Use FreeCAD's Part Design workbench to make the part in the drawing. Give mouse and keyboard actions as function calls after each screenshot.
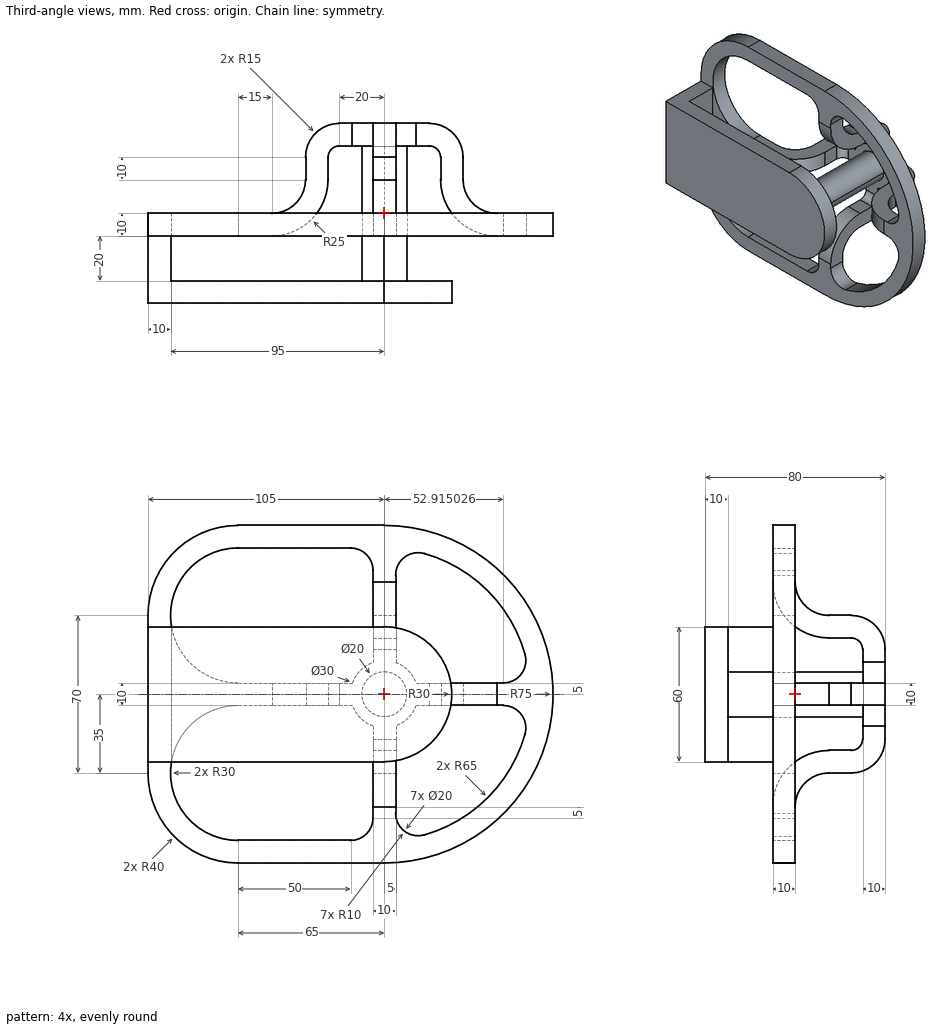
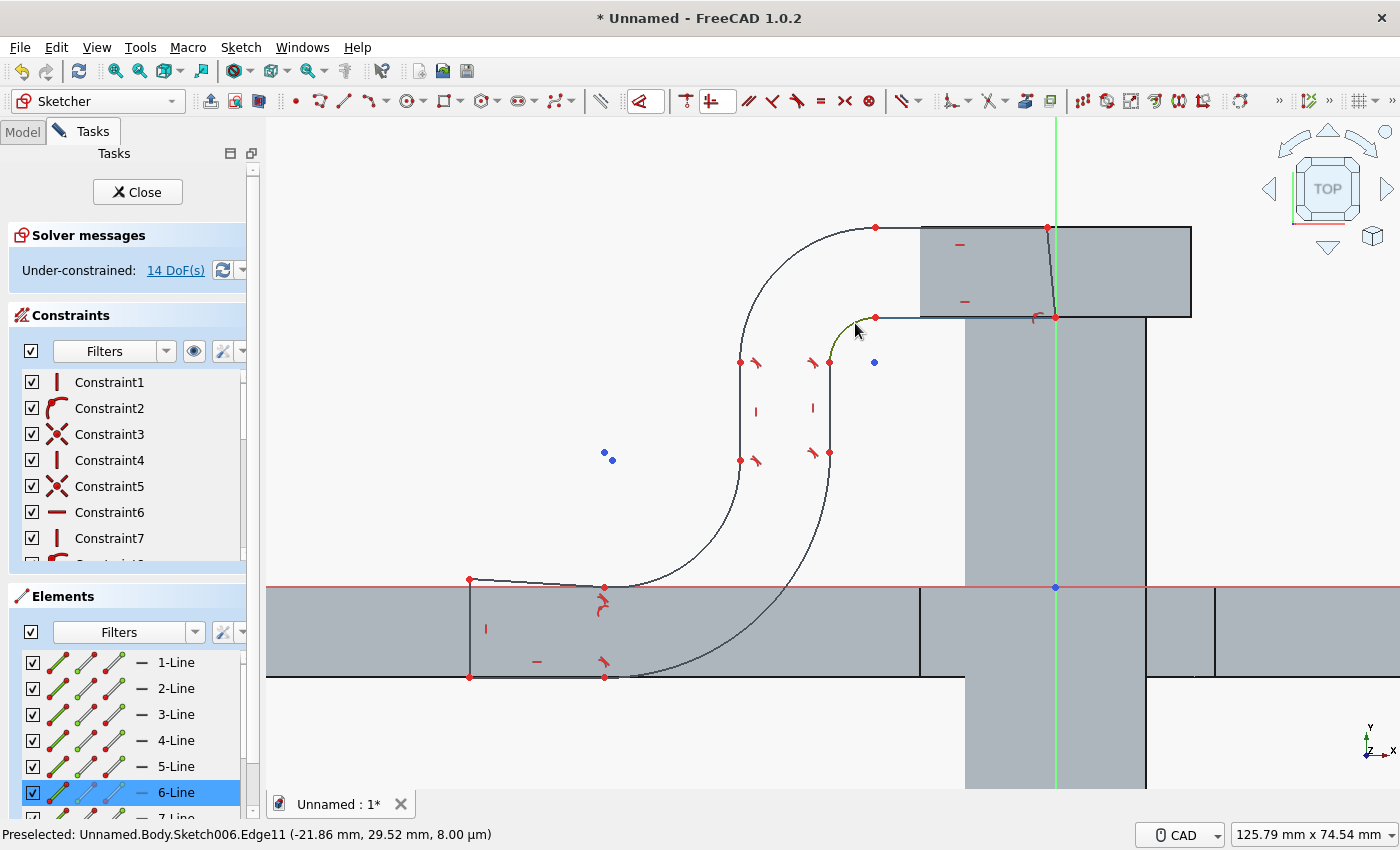
click(798, 102)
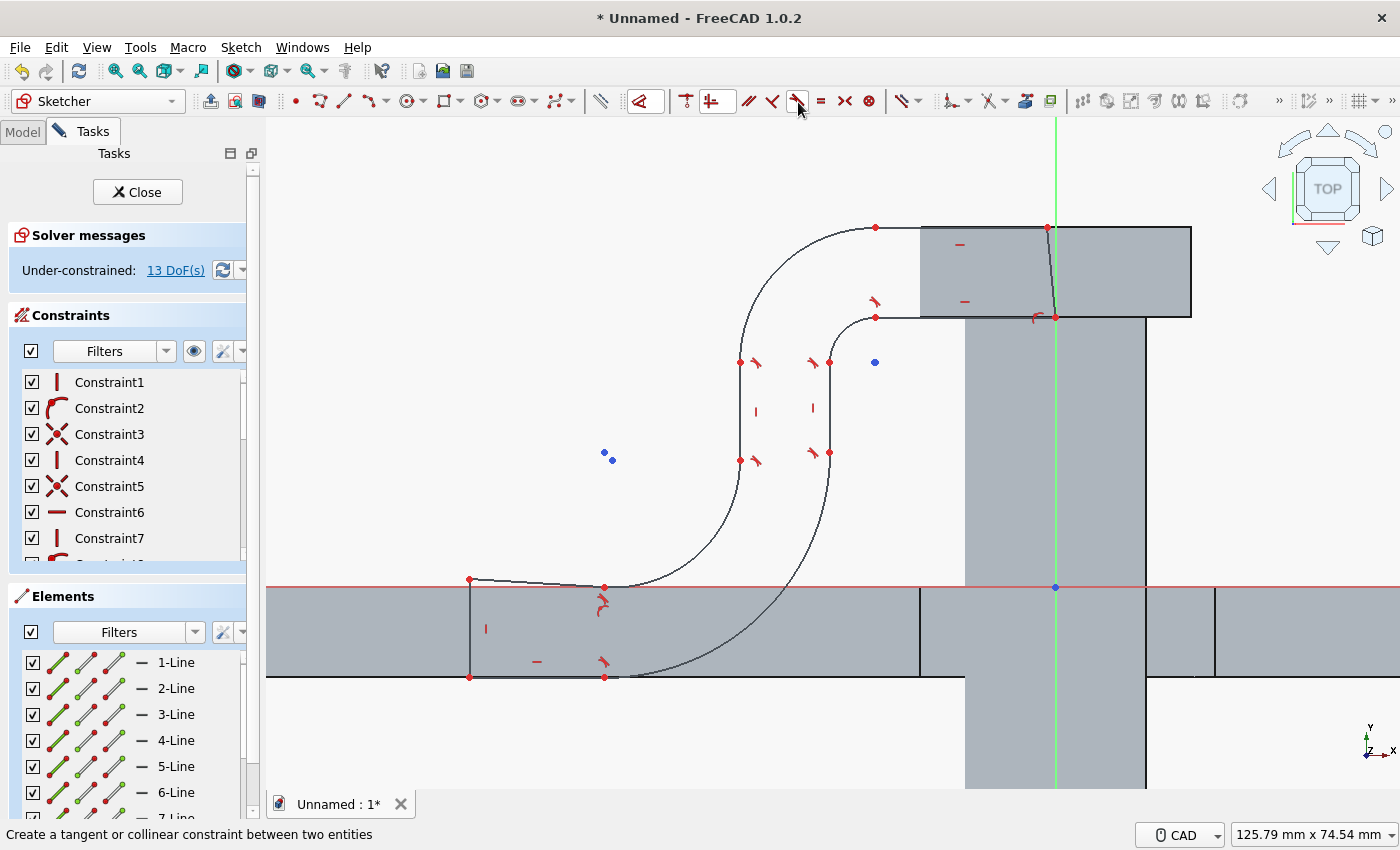
click(995, 228)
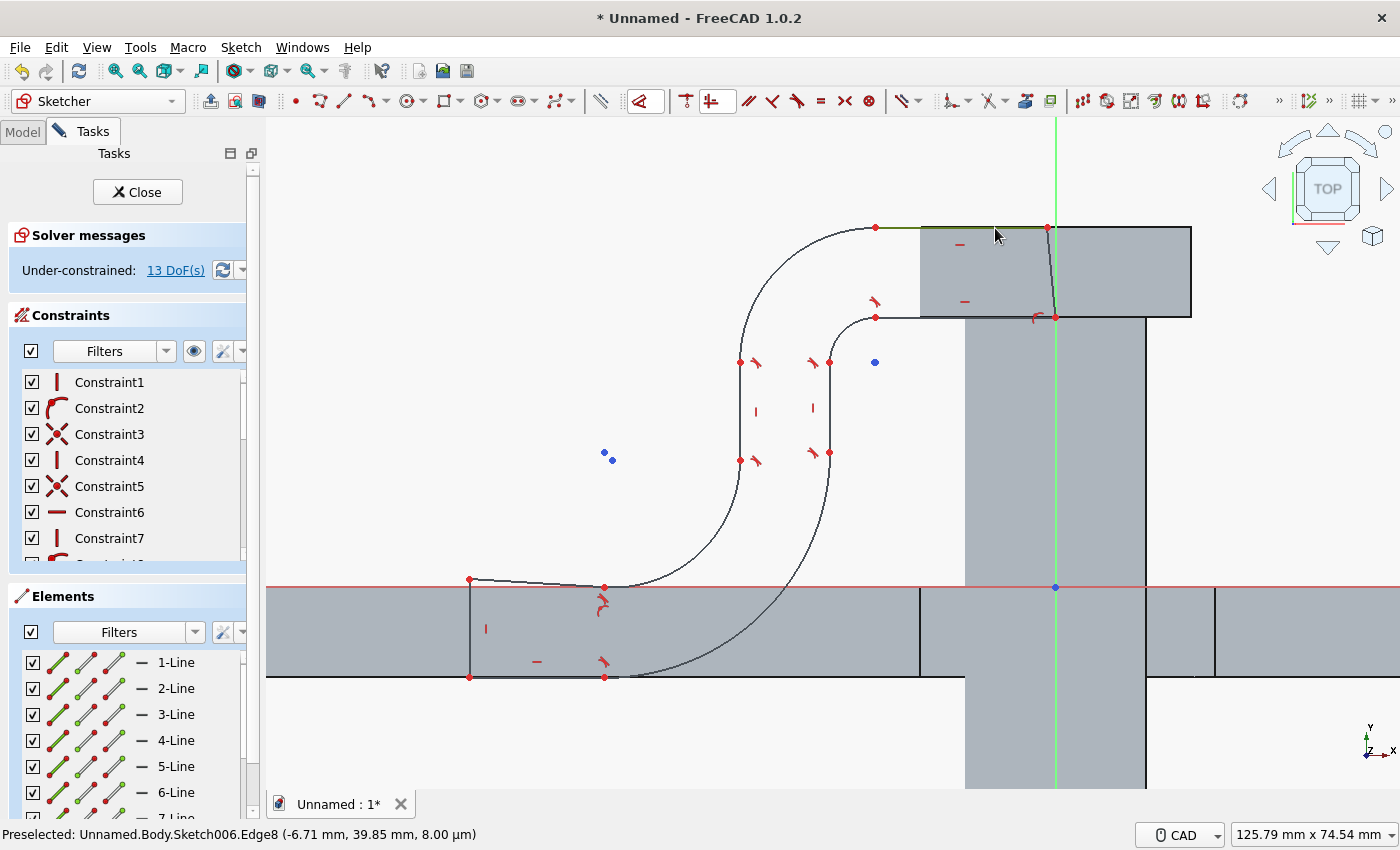
click(814, 243)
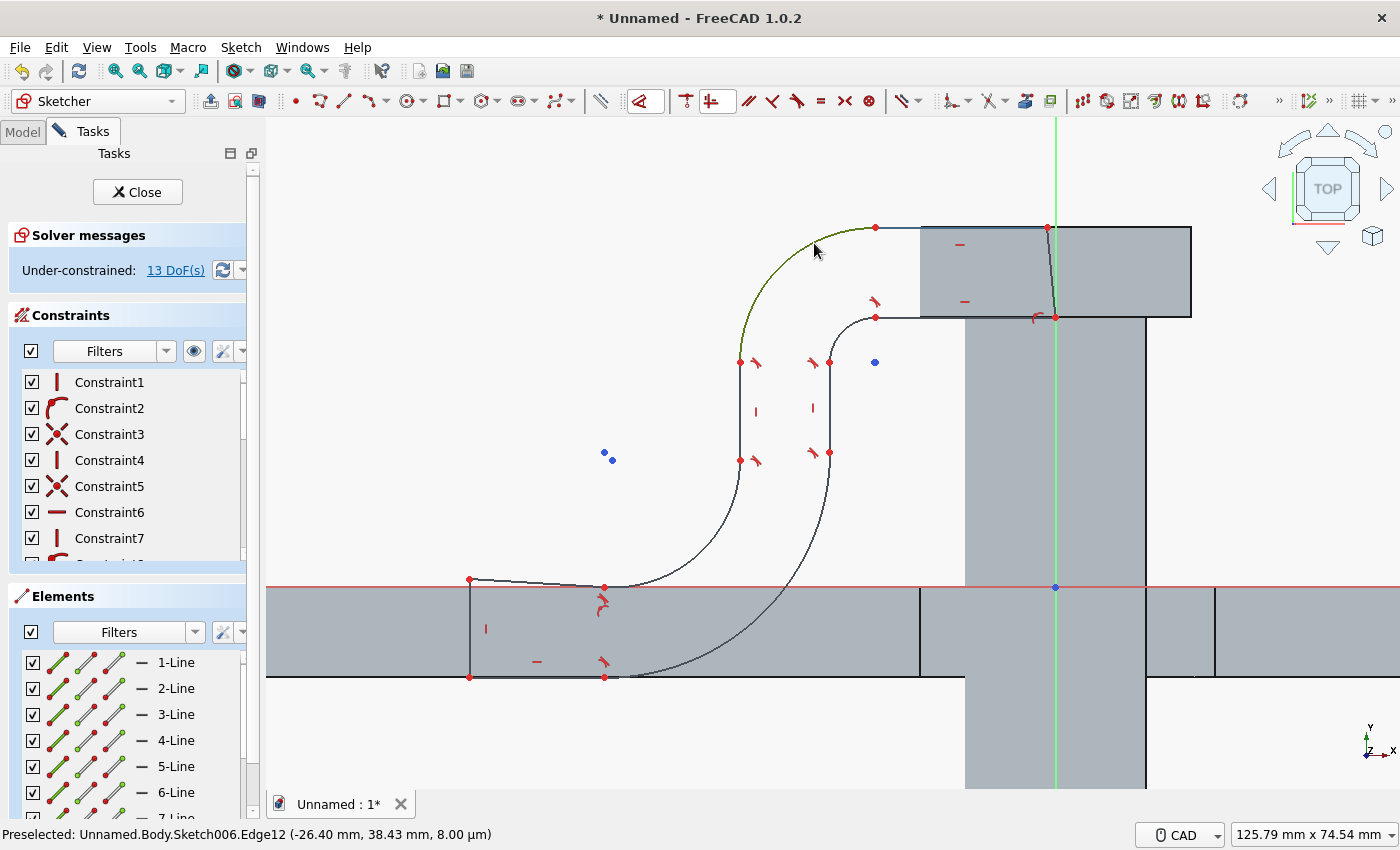
click(798, 102)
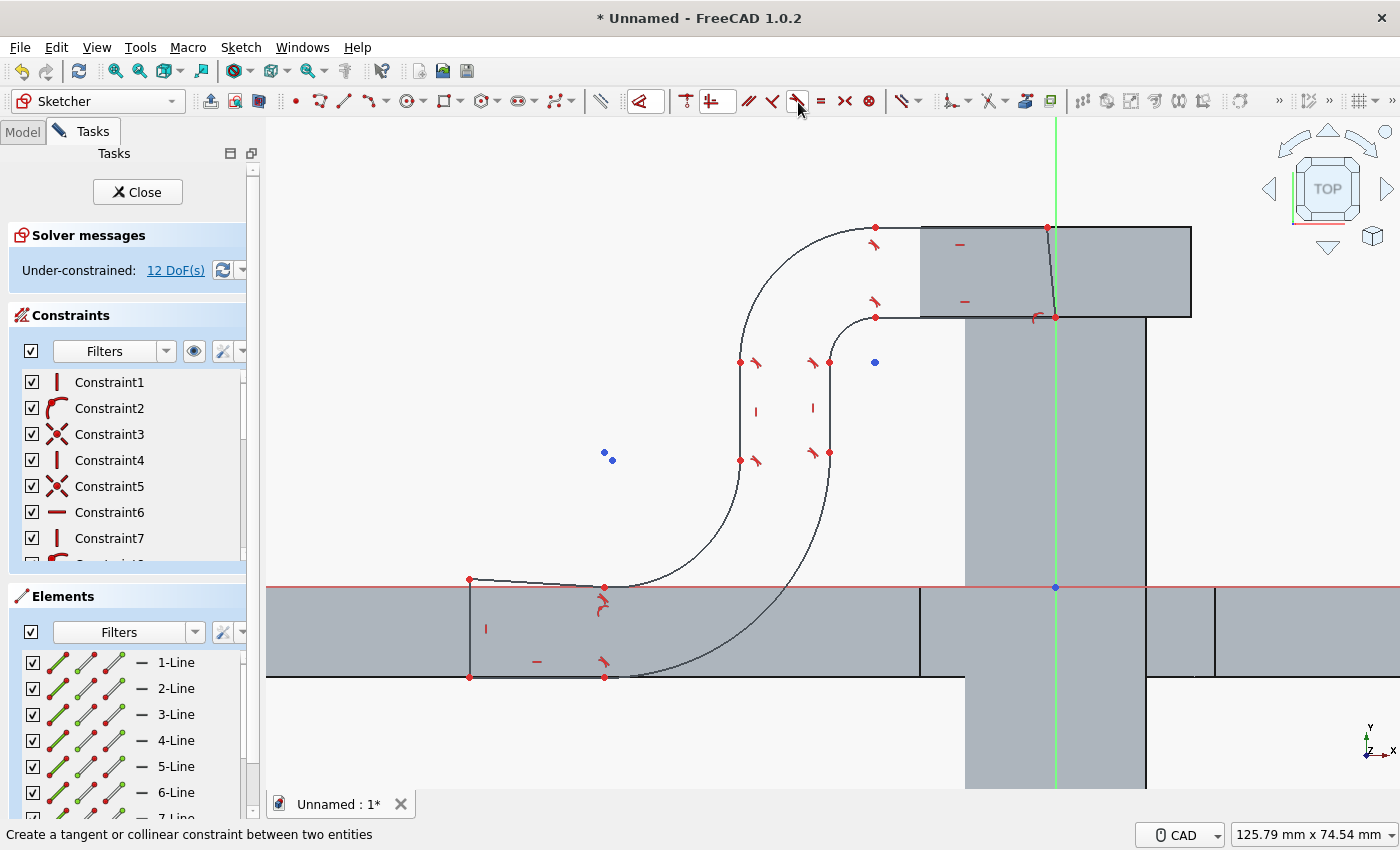
click(564, 585)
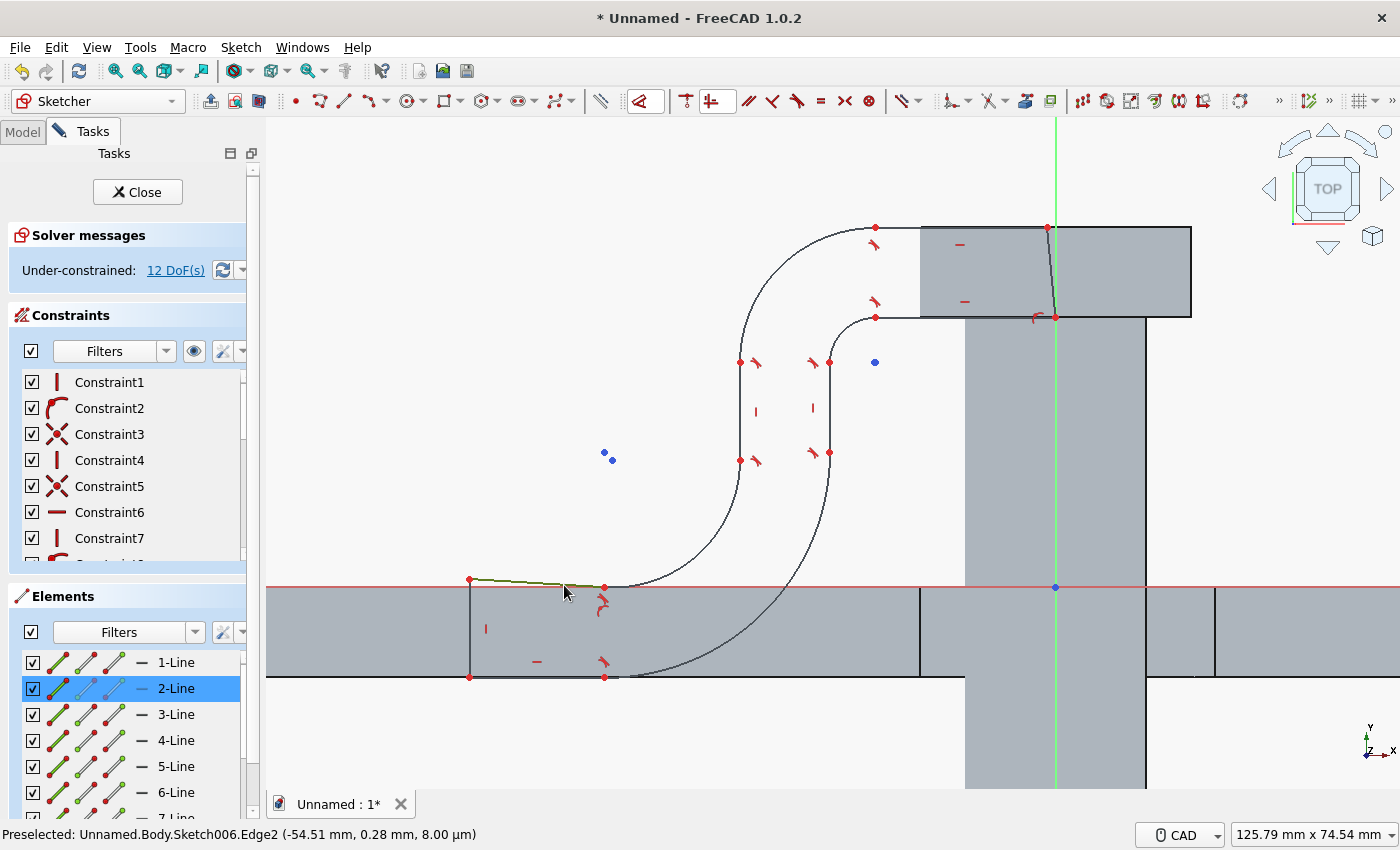
click(730, 102)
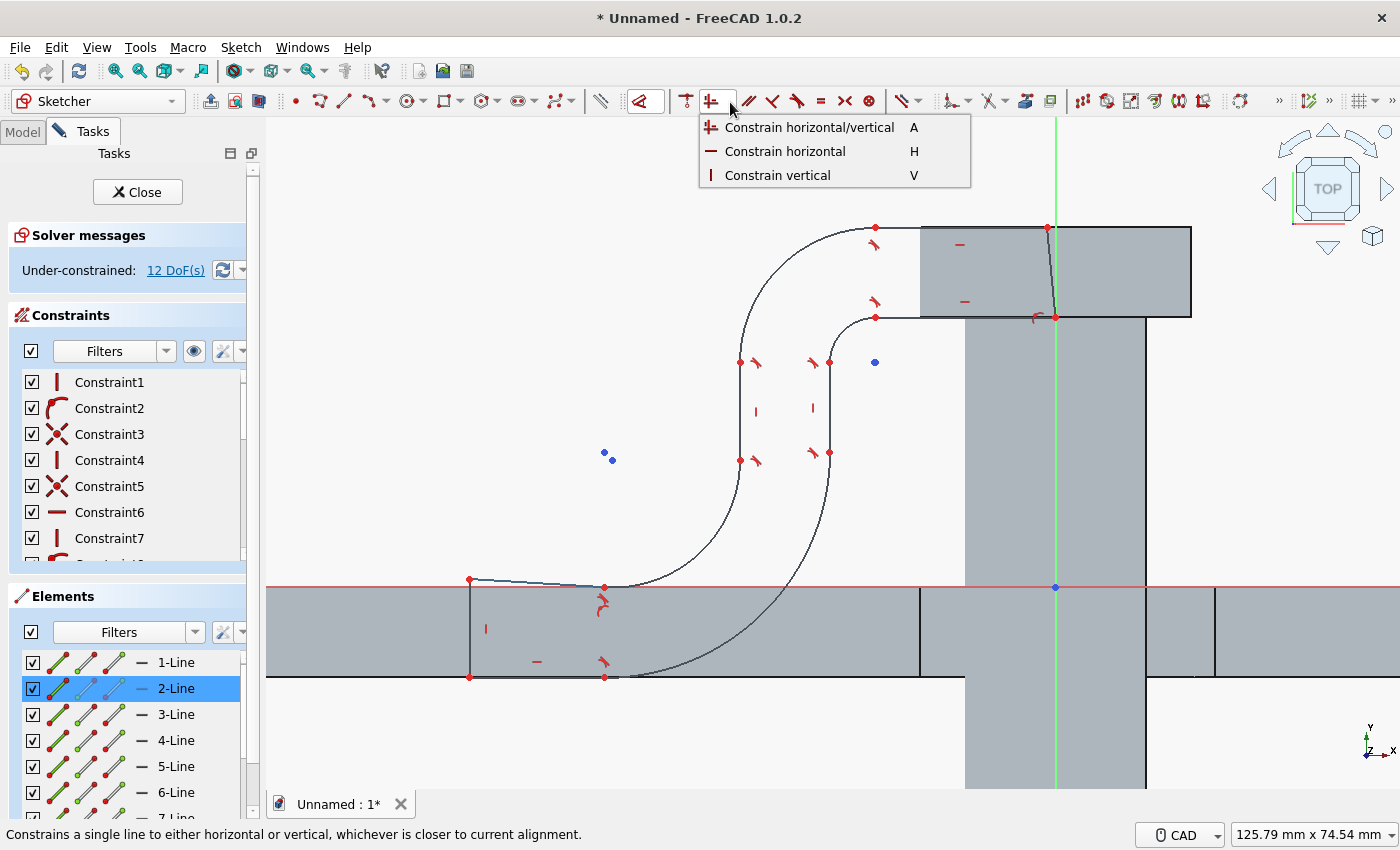
click(835, 151)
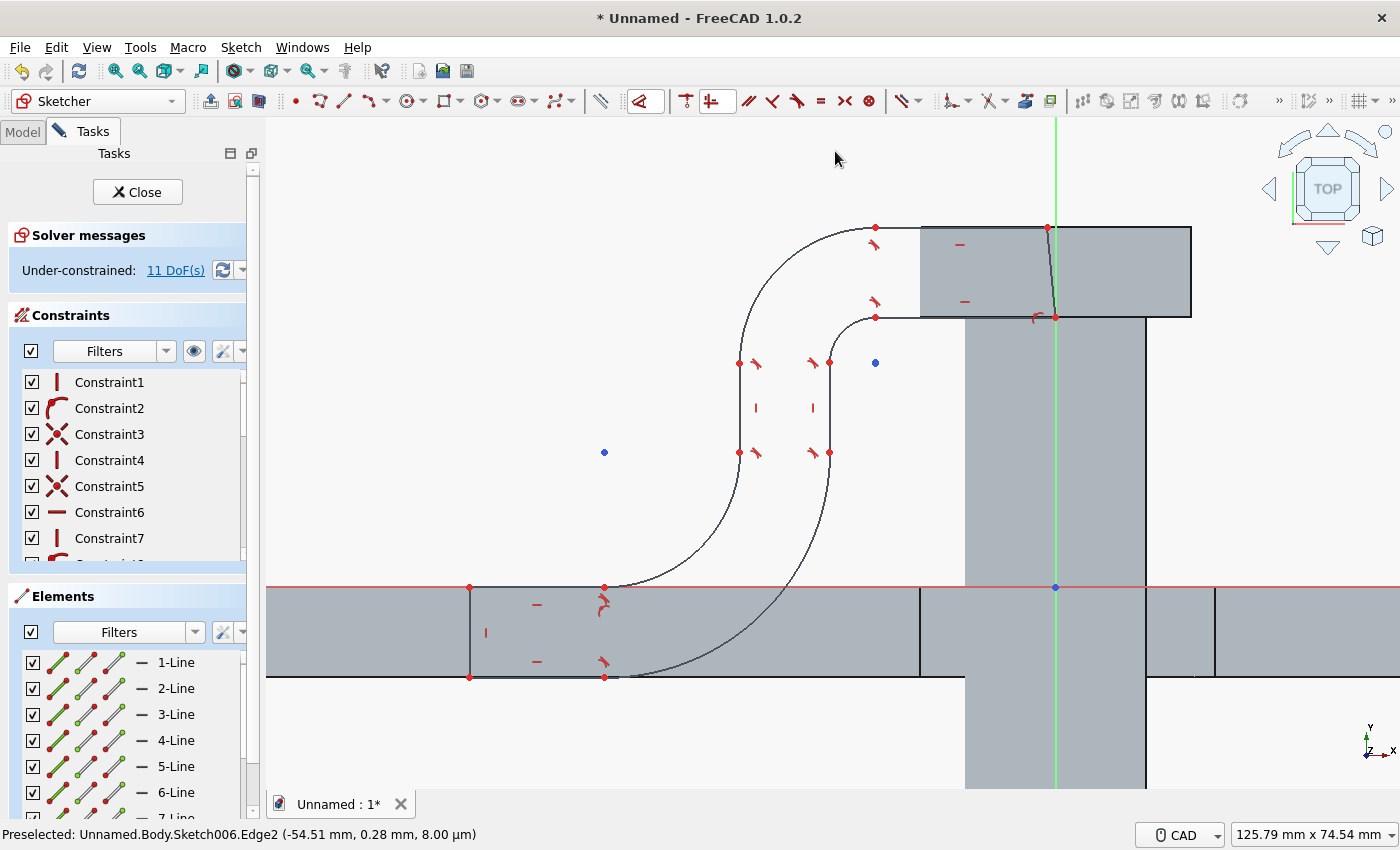
click(1053, 291)